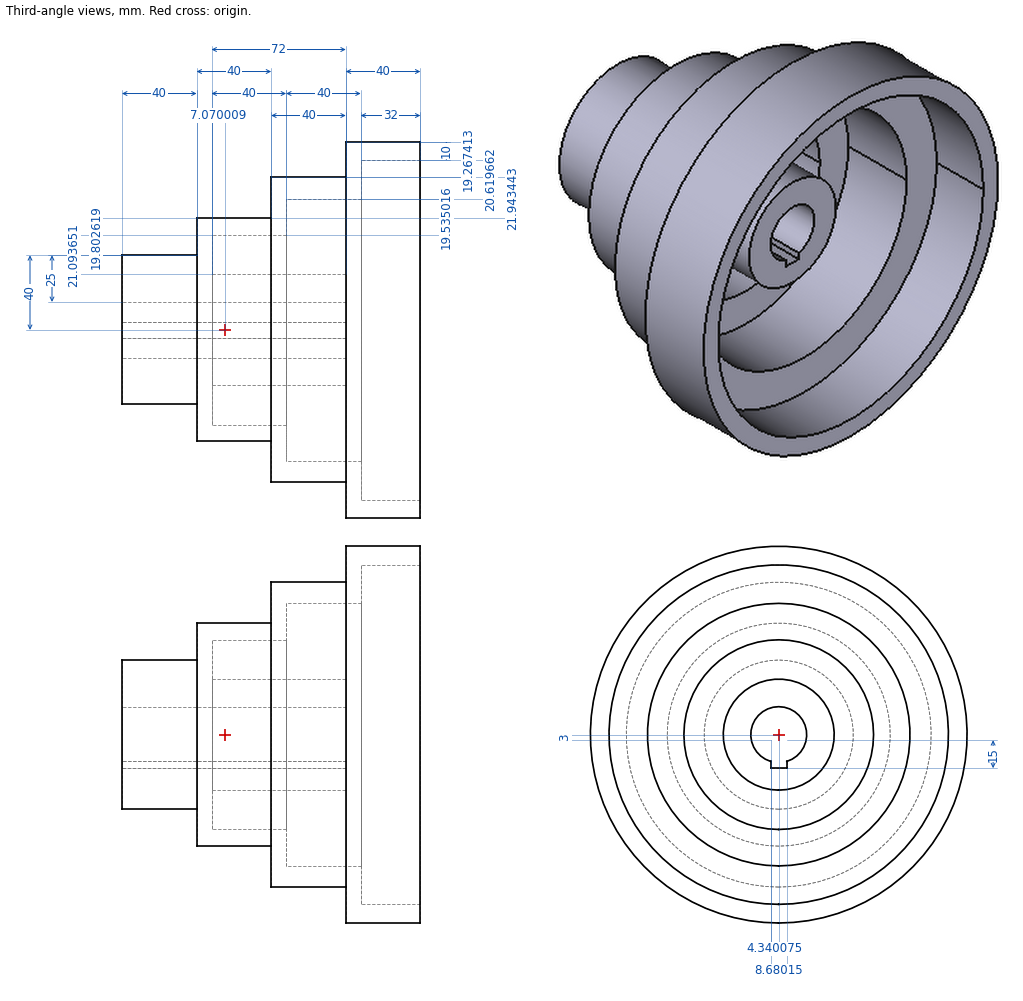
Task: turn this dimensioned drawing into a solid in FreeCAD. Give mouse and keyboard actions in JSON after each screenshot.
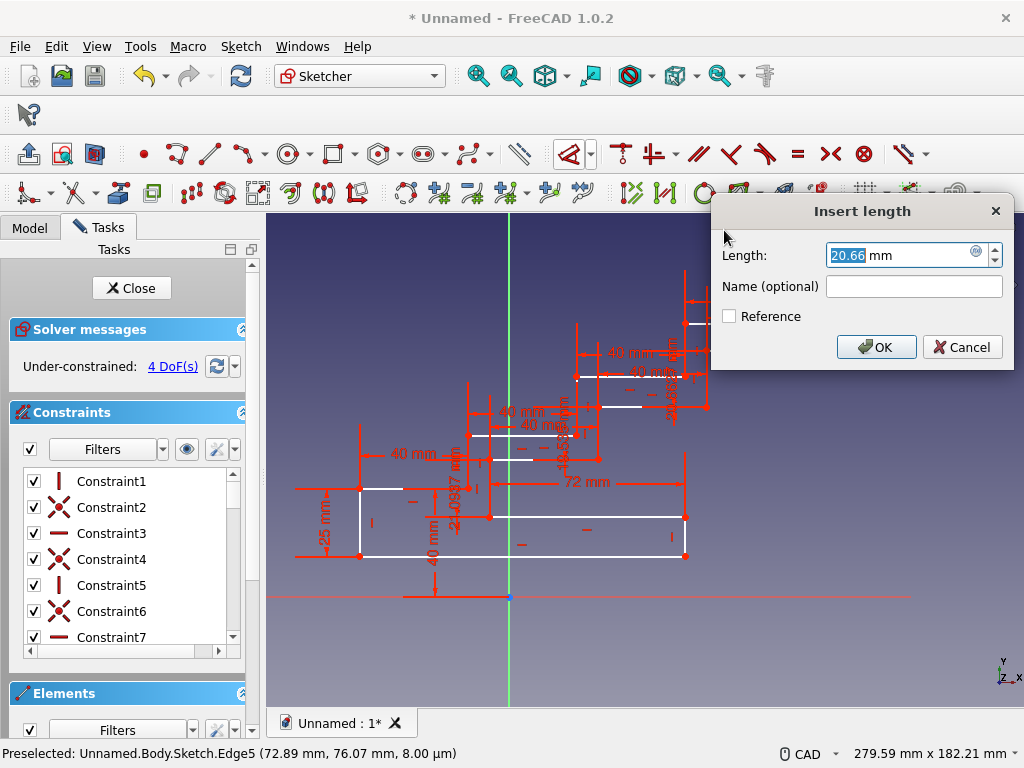
{"action": "type", "text": "20.619662"}
{"action": "key", "text": "Return"}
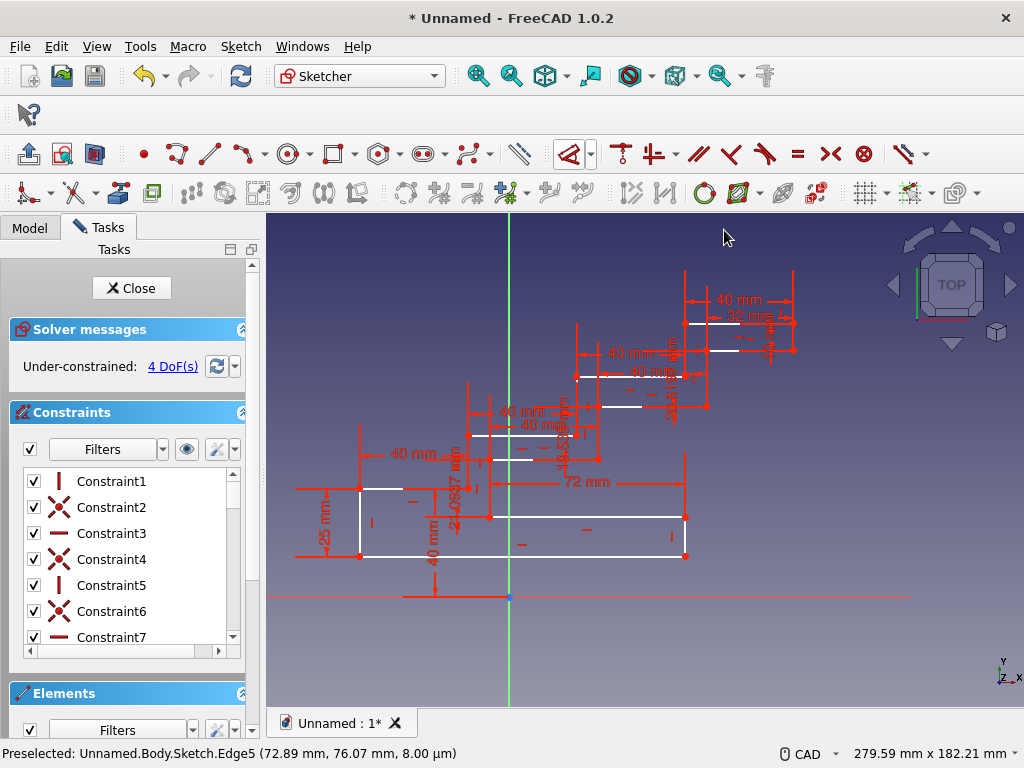
{"action": "left_click", "coordinate": [685, 340]}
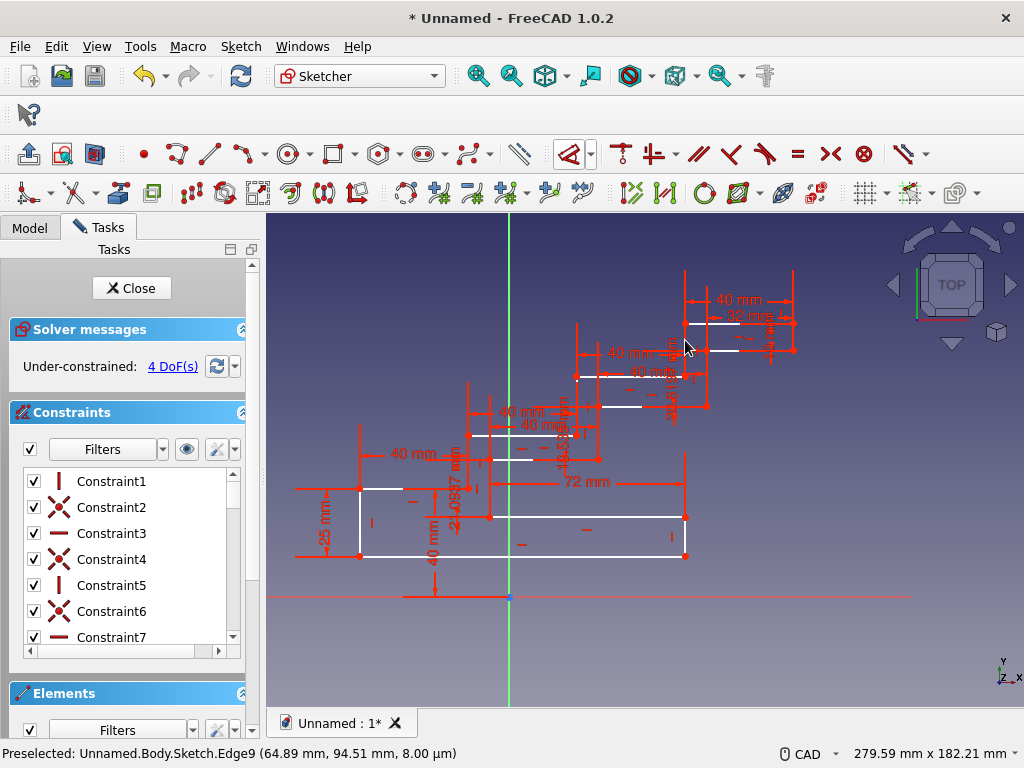
{"action": "key", "text": "i"}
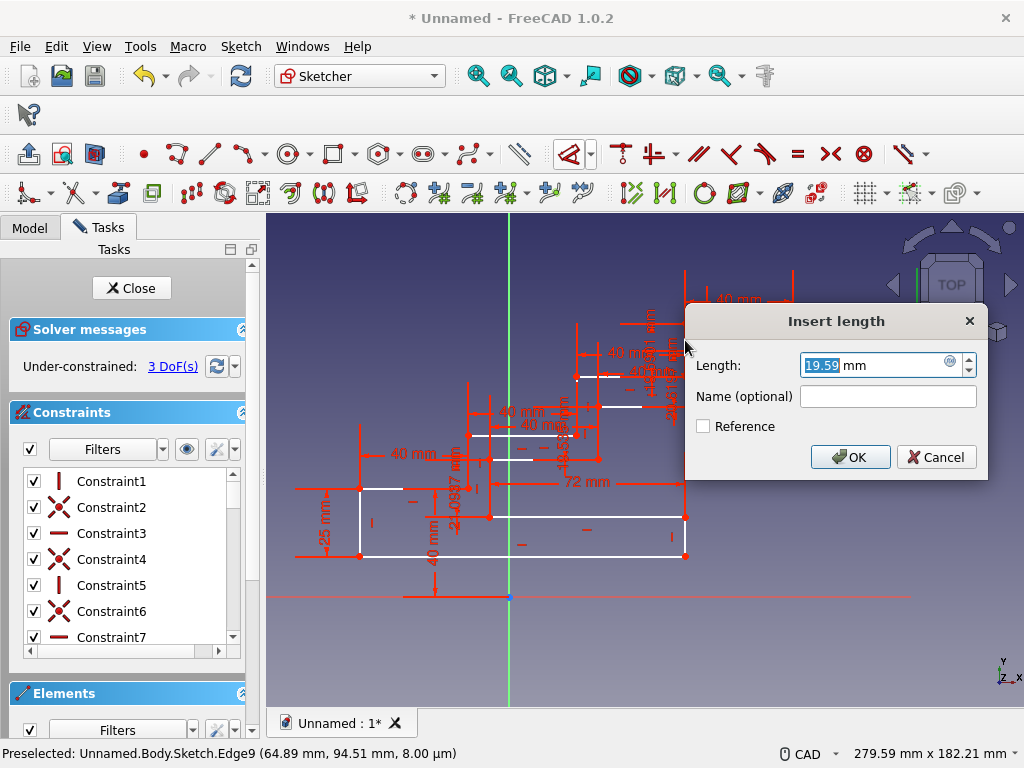
{"action": "type", "text": "19.267413"}
{"action": "key", "text": "Return"}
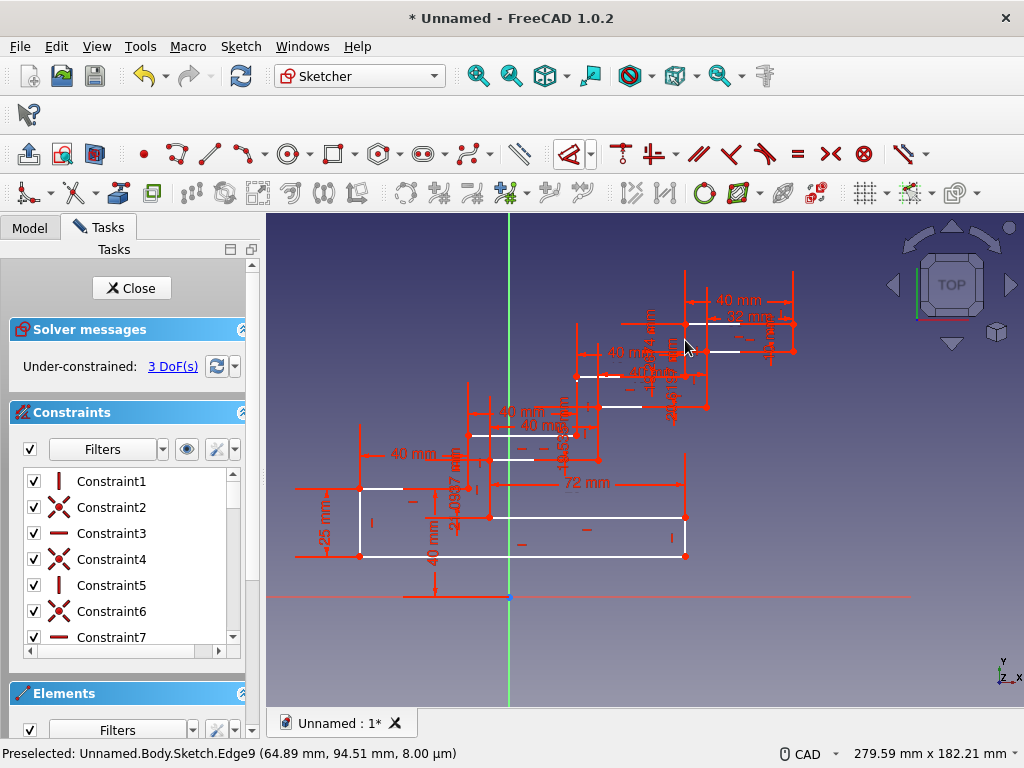
{"action": "left_click", "coordinate": [577, 394]}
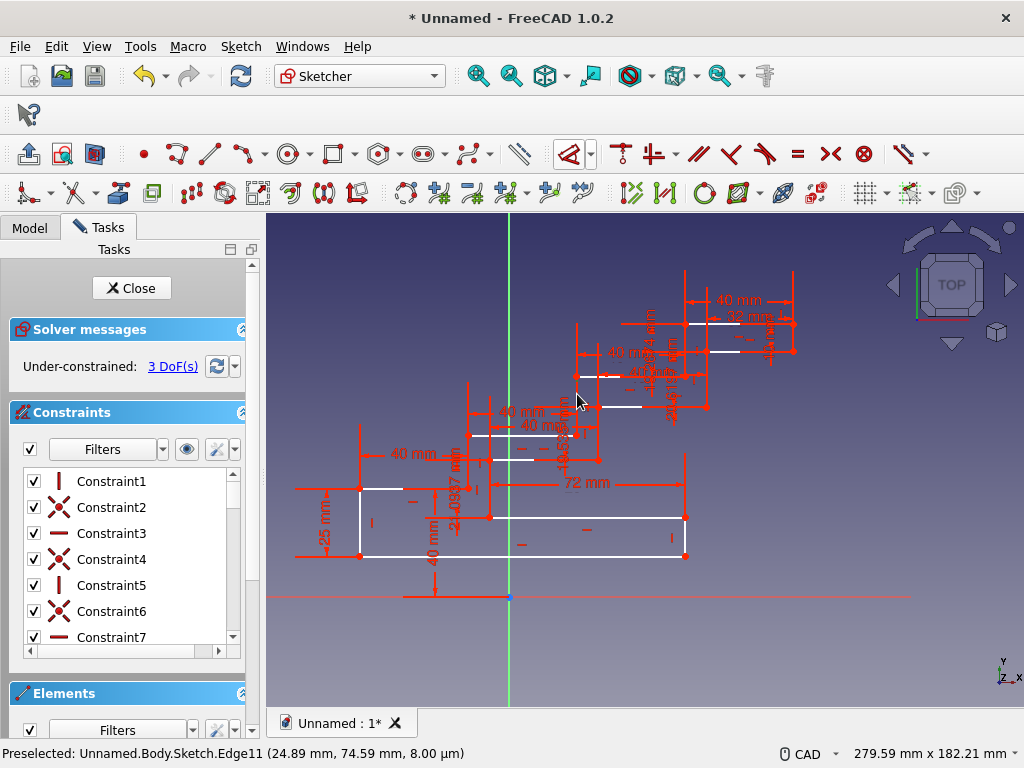
{"action": "key", "text": "i"}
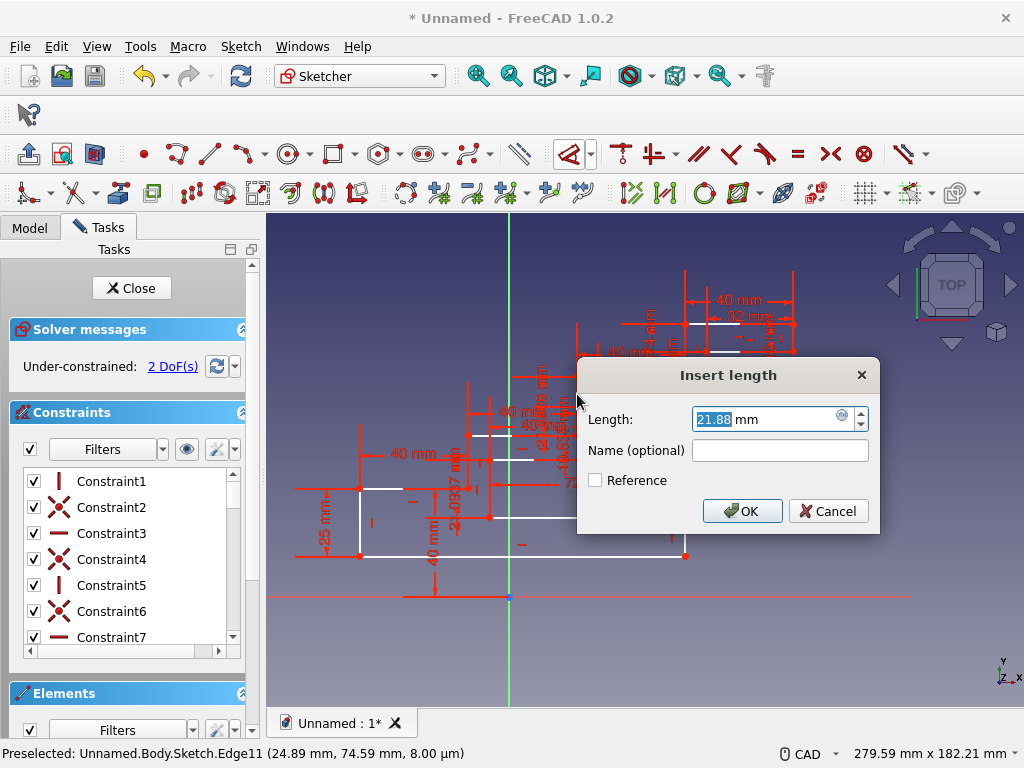
{"action": "type", "text": "21.943443"}
{"action": "key", "text": "Return"}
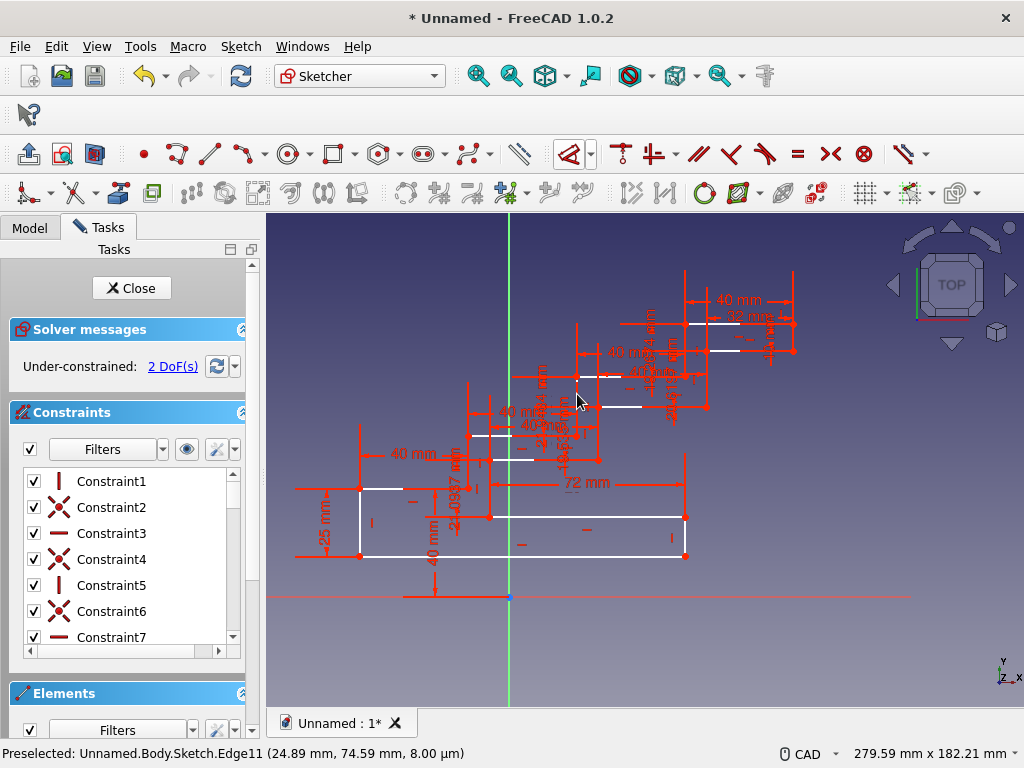
{"action": "left_click", "coordinate": [468, 452]}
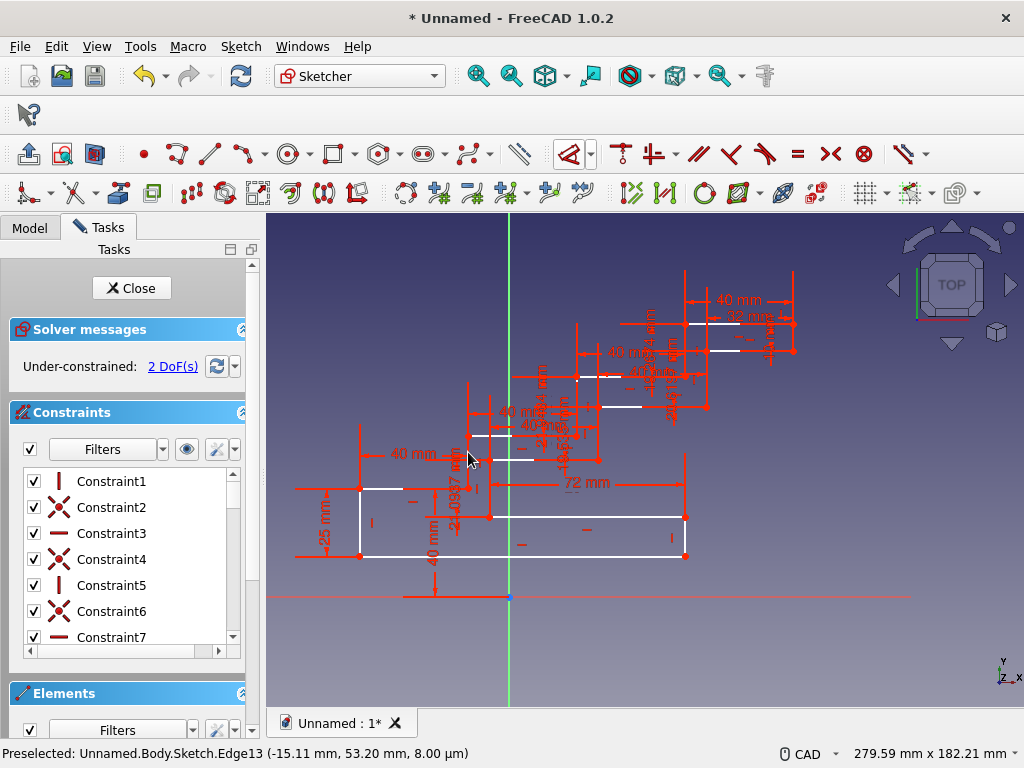
{"action": "key", "text": "i"}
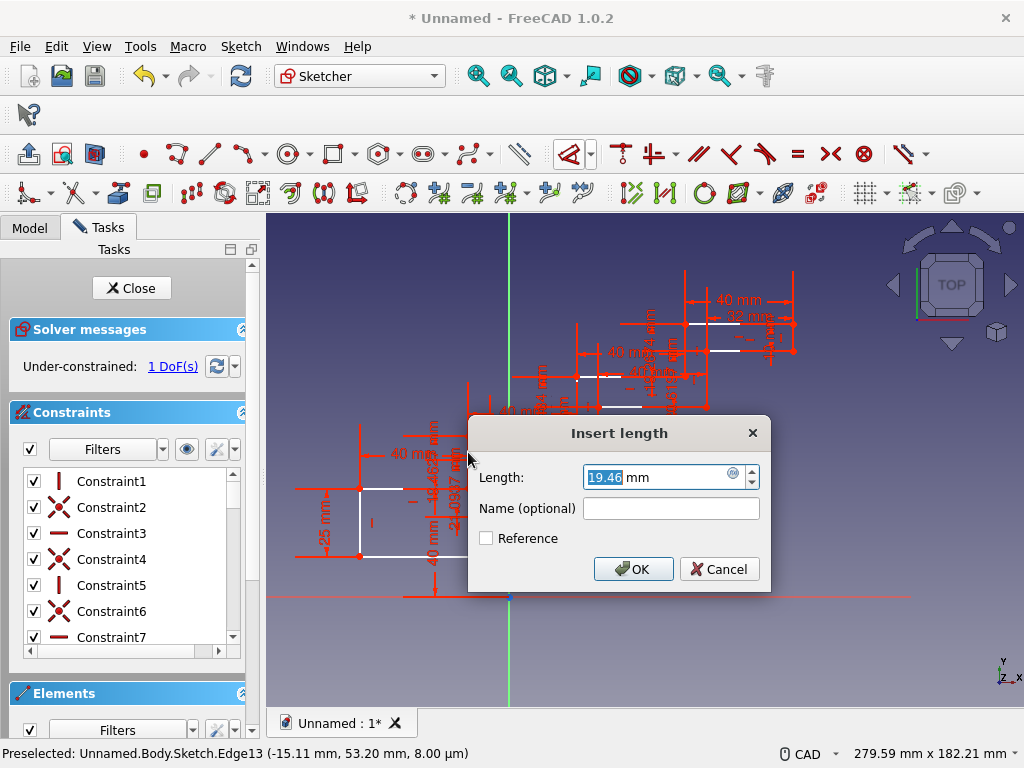
{"action": "type", "text": "19.802619"}
{"action": "key", "text": "Return"}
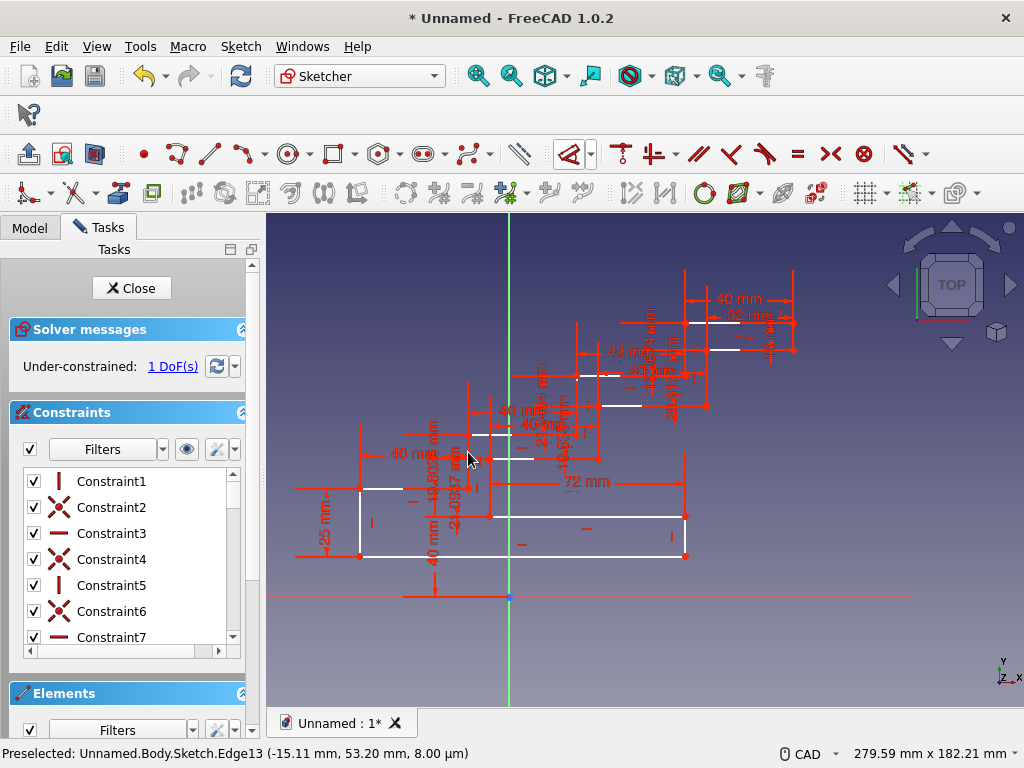
{"action": "scroll", "coordinate": [490, 517], "scroll_direction": "up", "scroll_amount": 4}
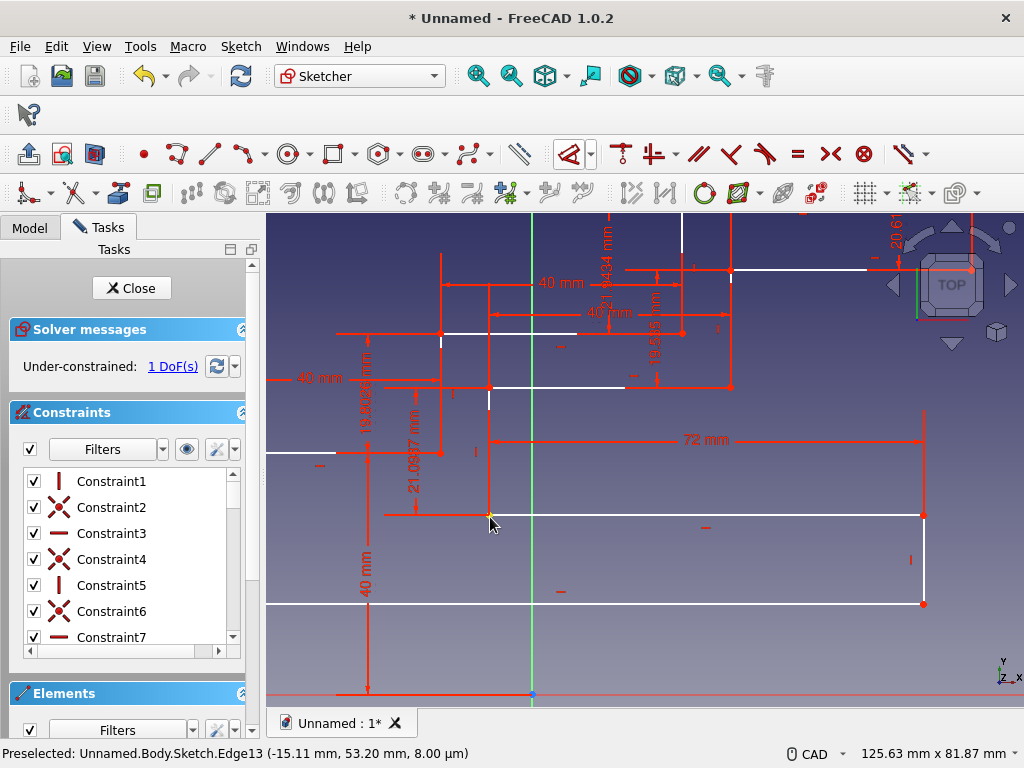
{"action": "left_click", "coordinate": [489, 515]}